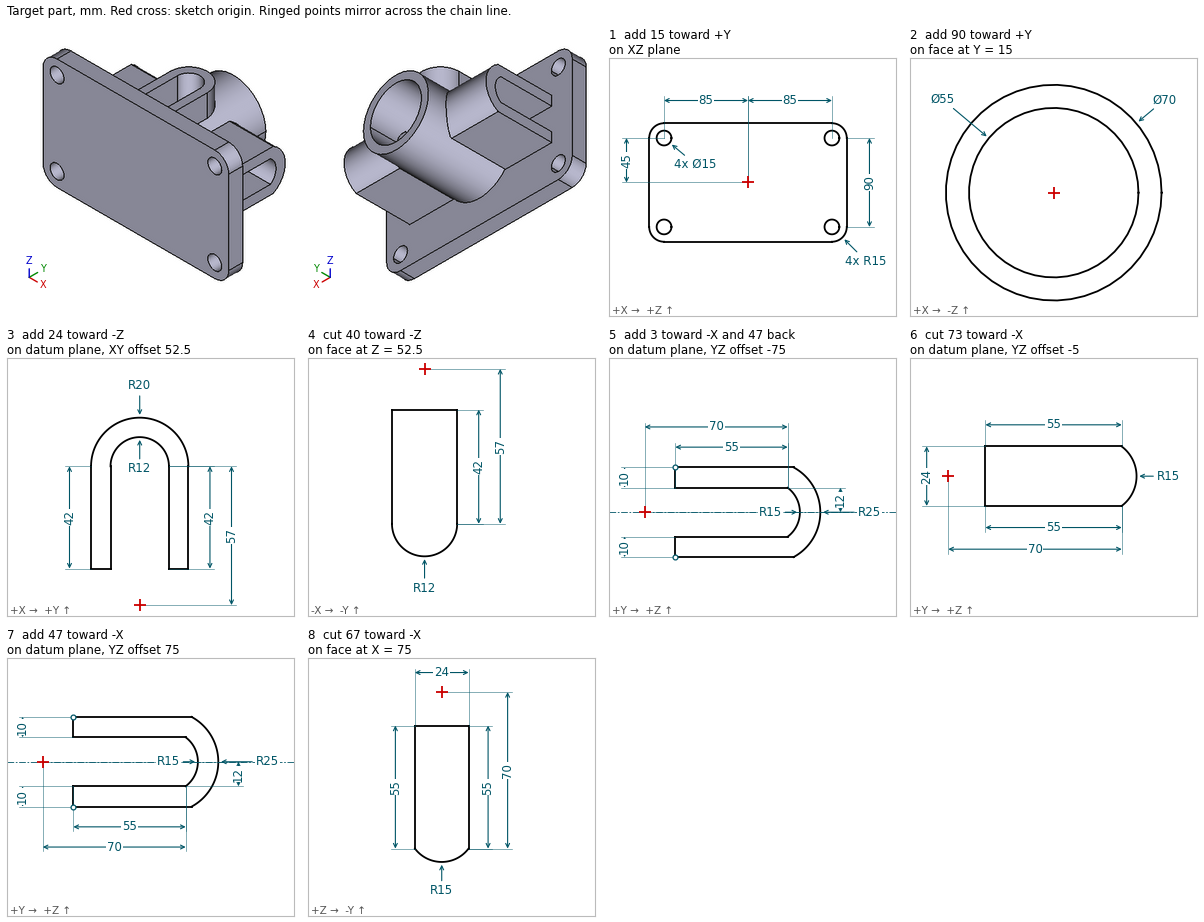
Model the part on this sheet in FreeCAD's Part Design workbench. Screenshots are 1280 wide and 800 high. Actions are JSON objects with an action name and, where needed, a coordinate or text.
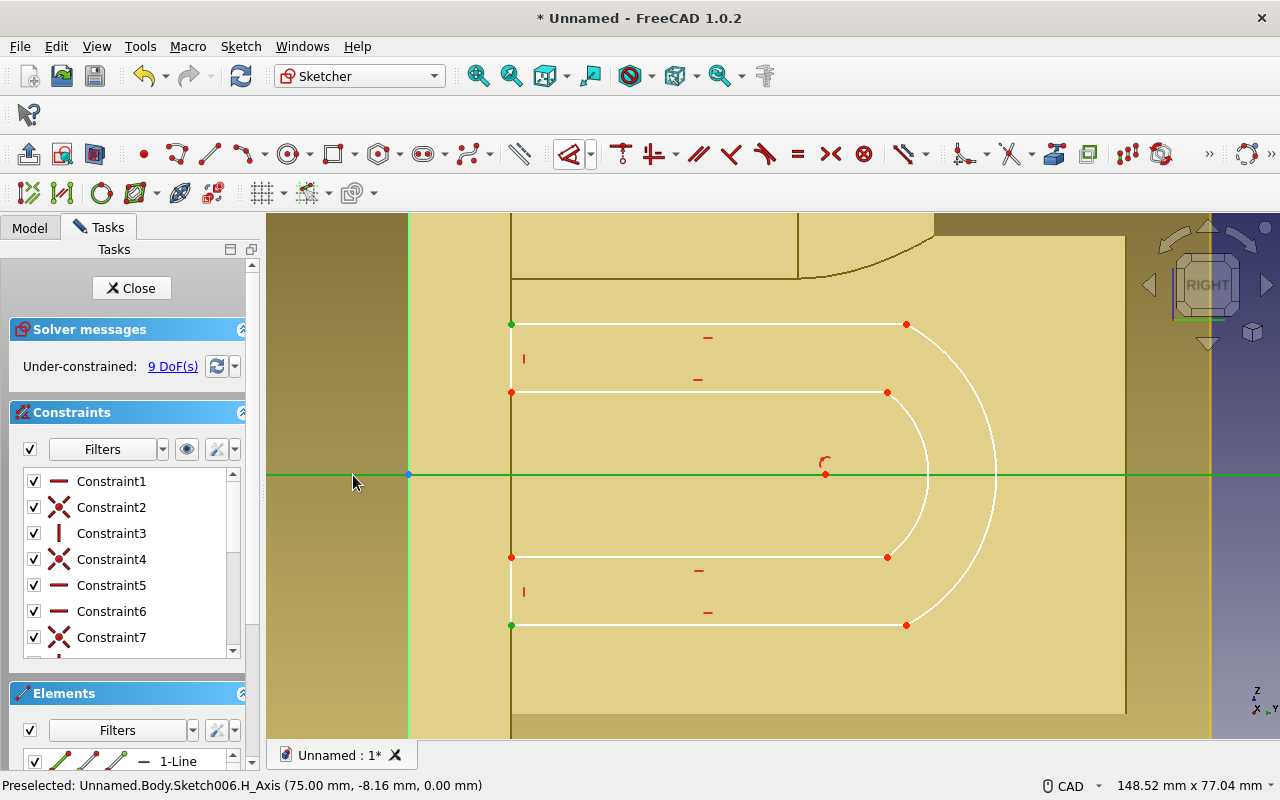
{"action": "key", "text": "s"}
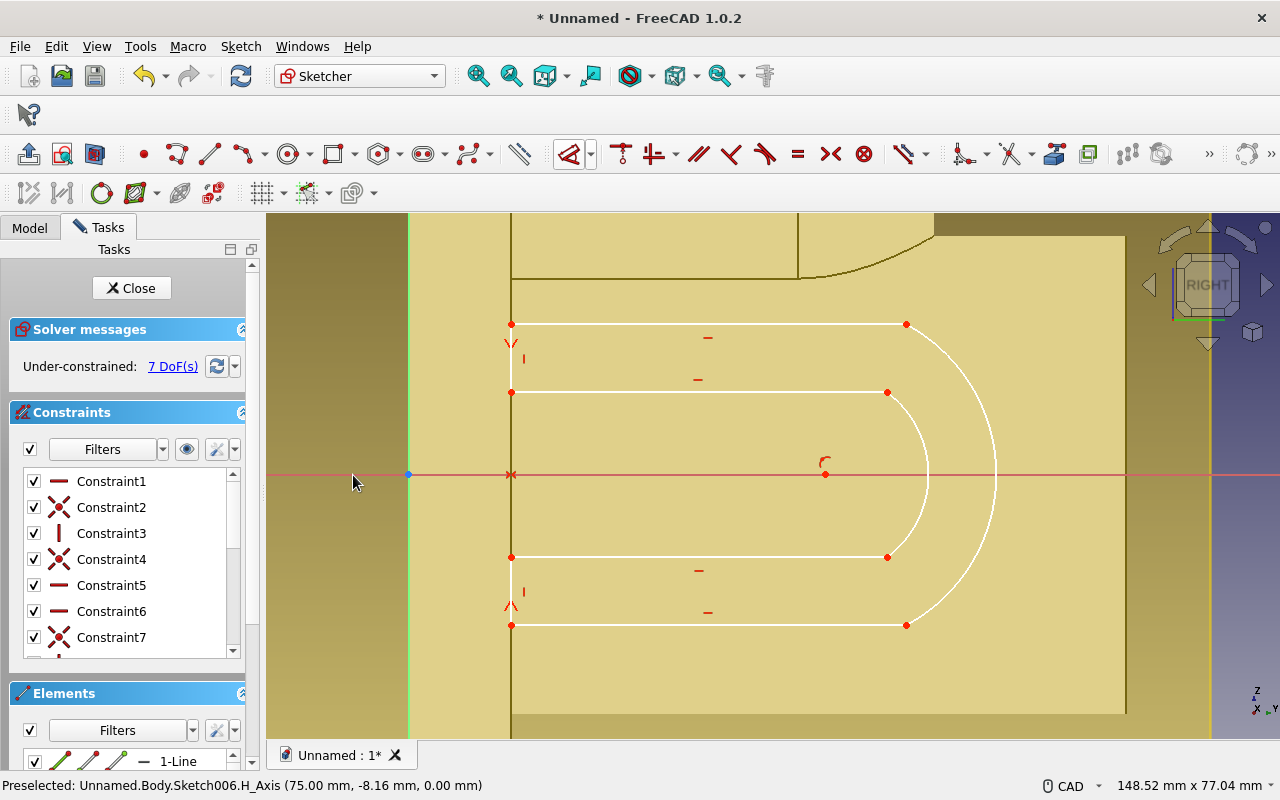
{"action": "left_click", "coordinate": [981, 546]}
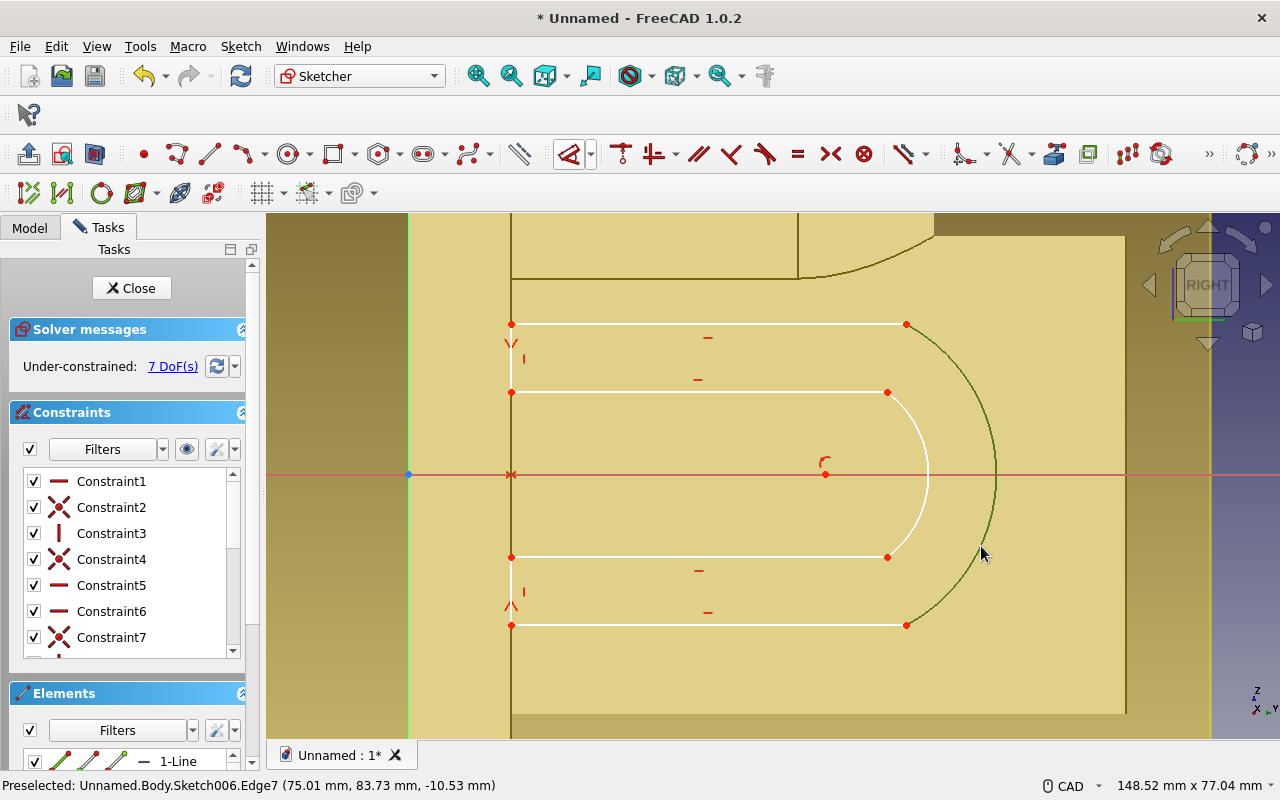
{"action": "left_click", "coordinate": [590, 154]}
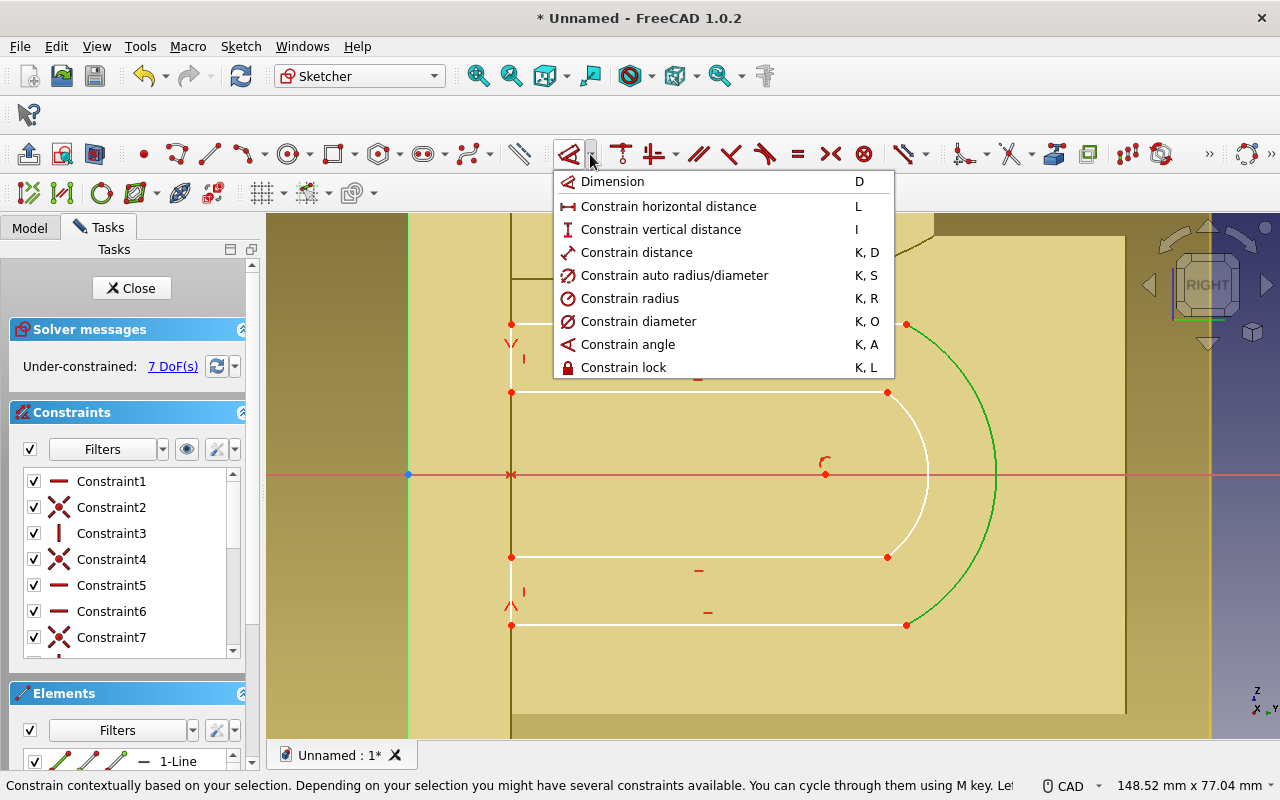
{"action": "left_click", "coordinate": [724, 298]}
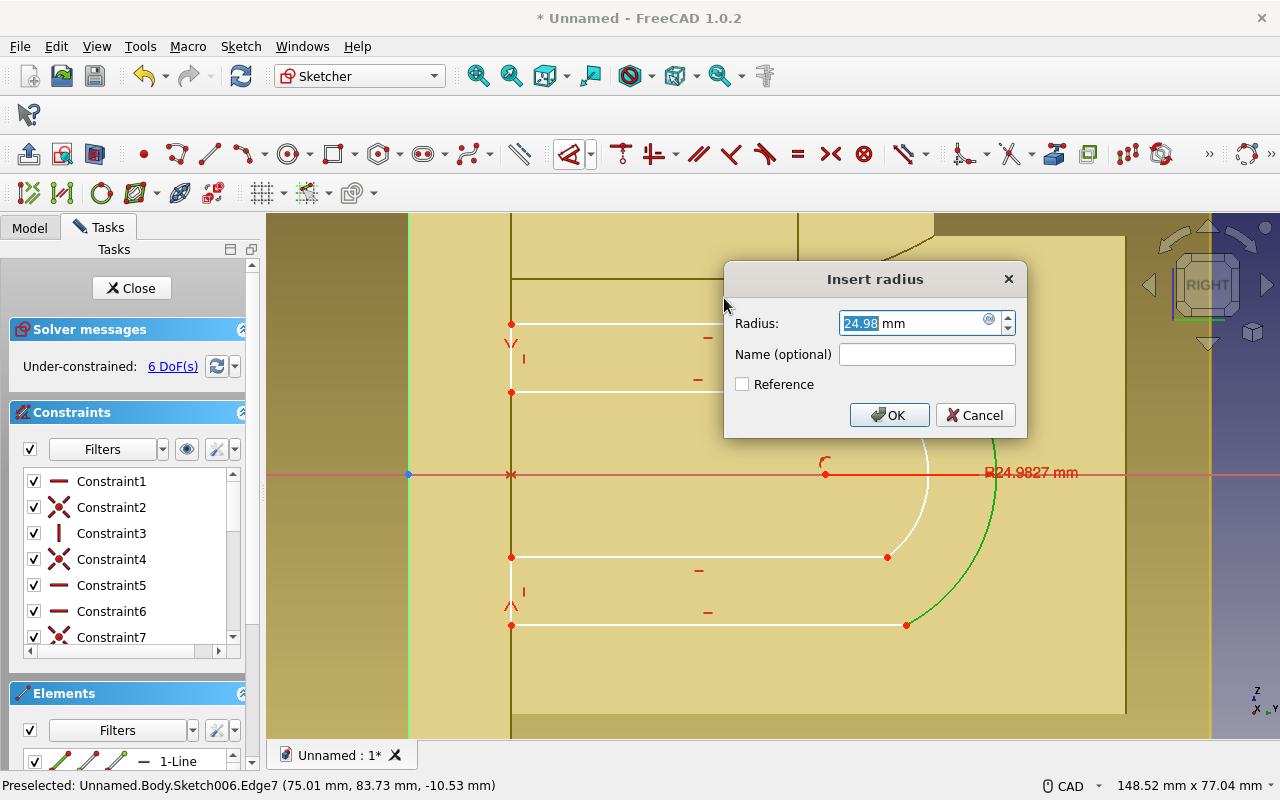
{"action": "type", "text": "25"}
{"action": "key", "text": "Return"}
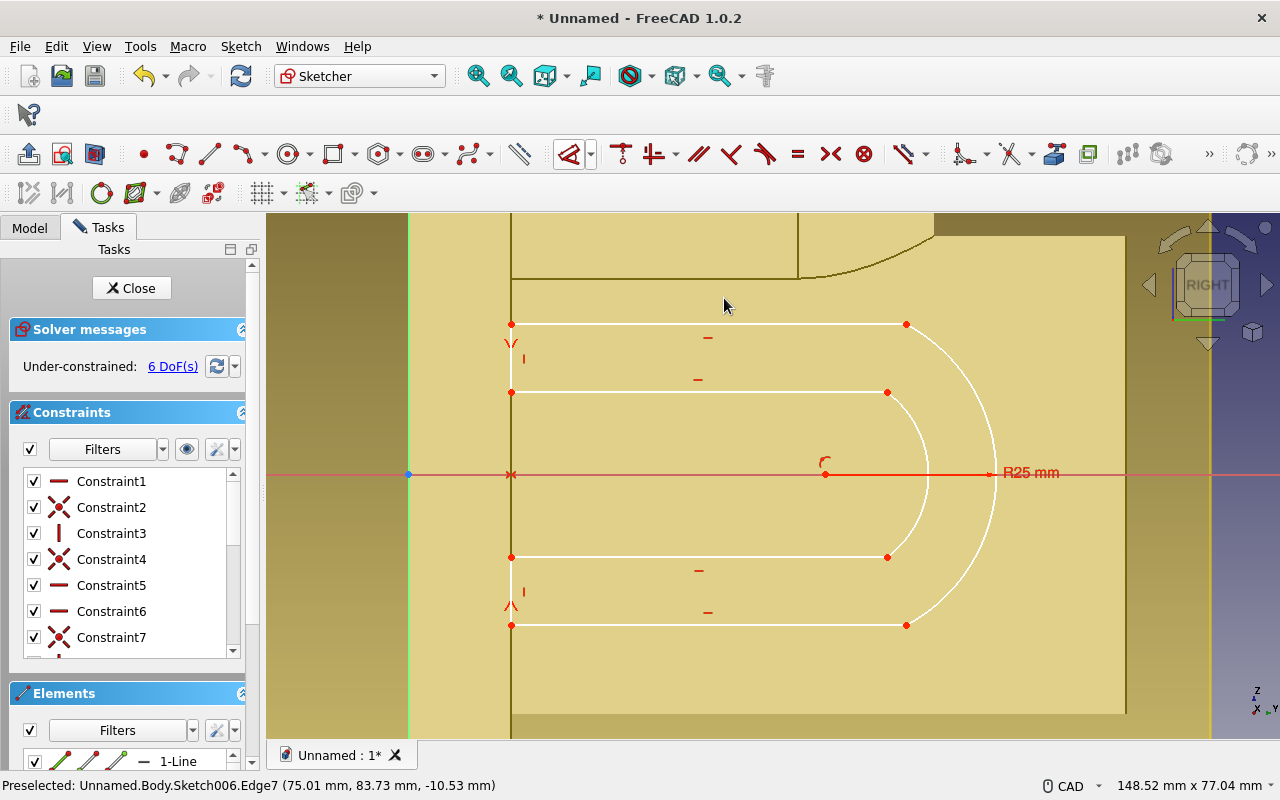
{"action": "left_click", "coordinate": [921, 512]}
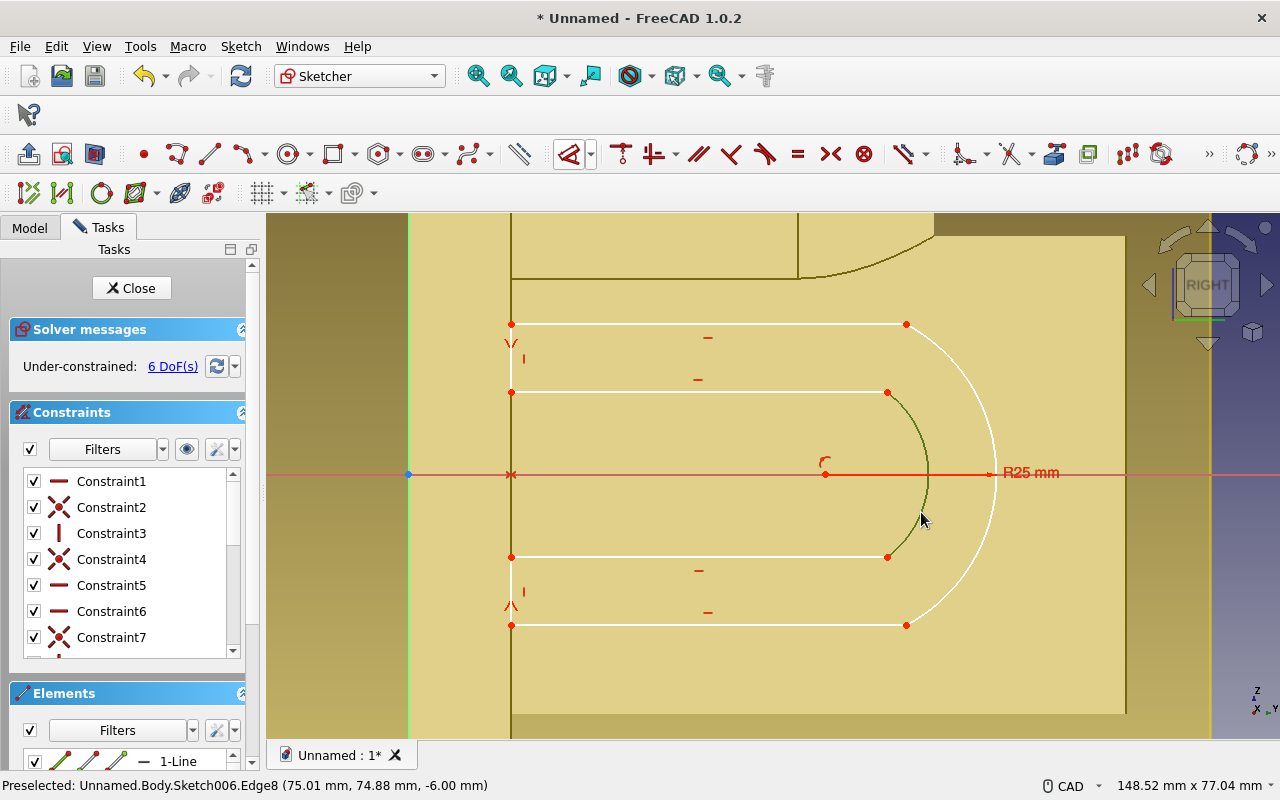
{"action": "key", "text": "k r"}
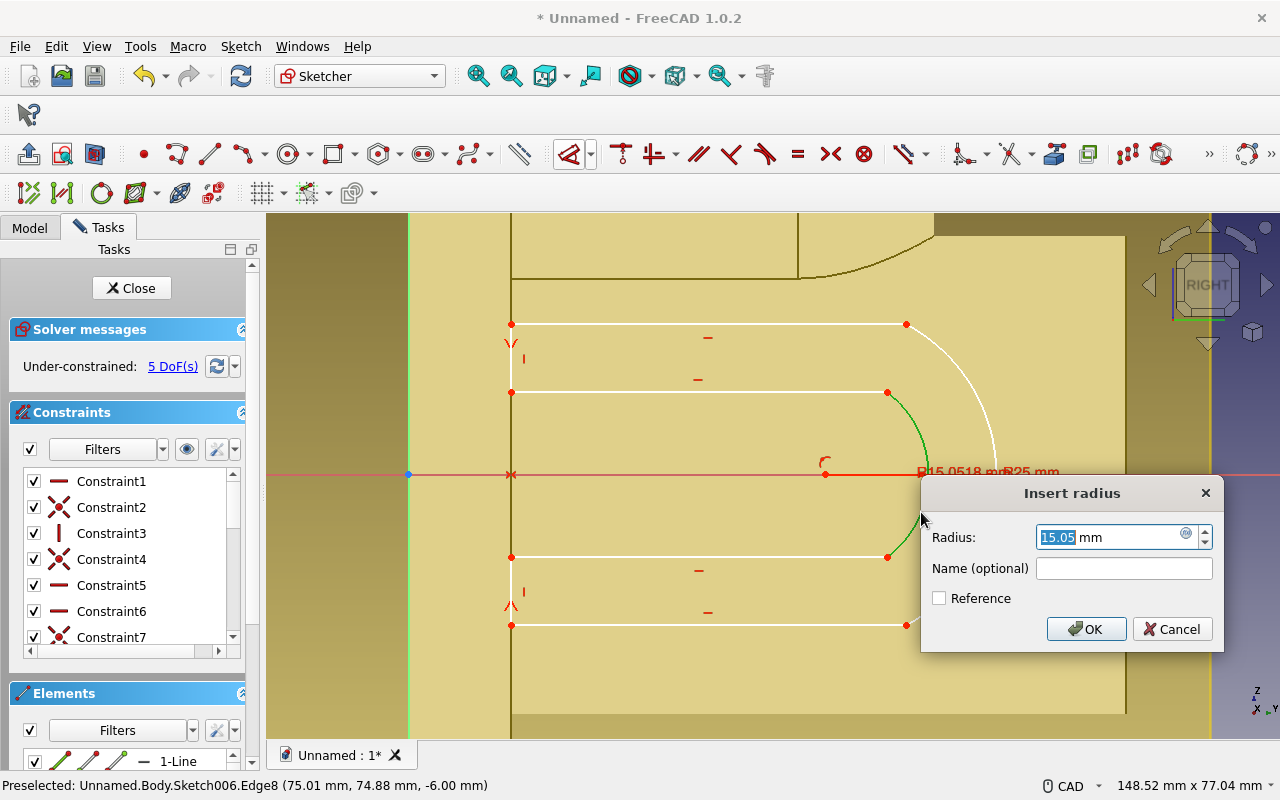
{"action": "type", "text": "15"}
{"action": "key", "text": "Return"}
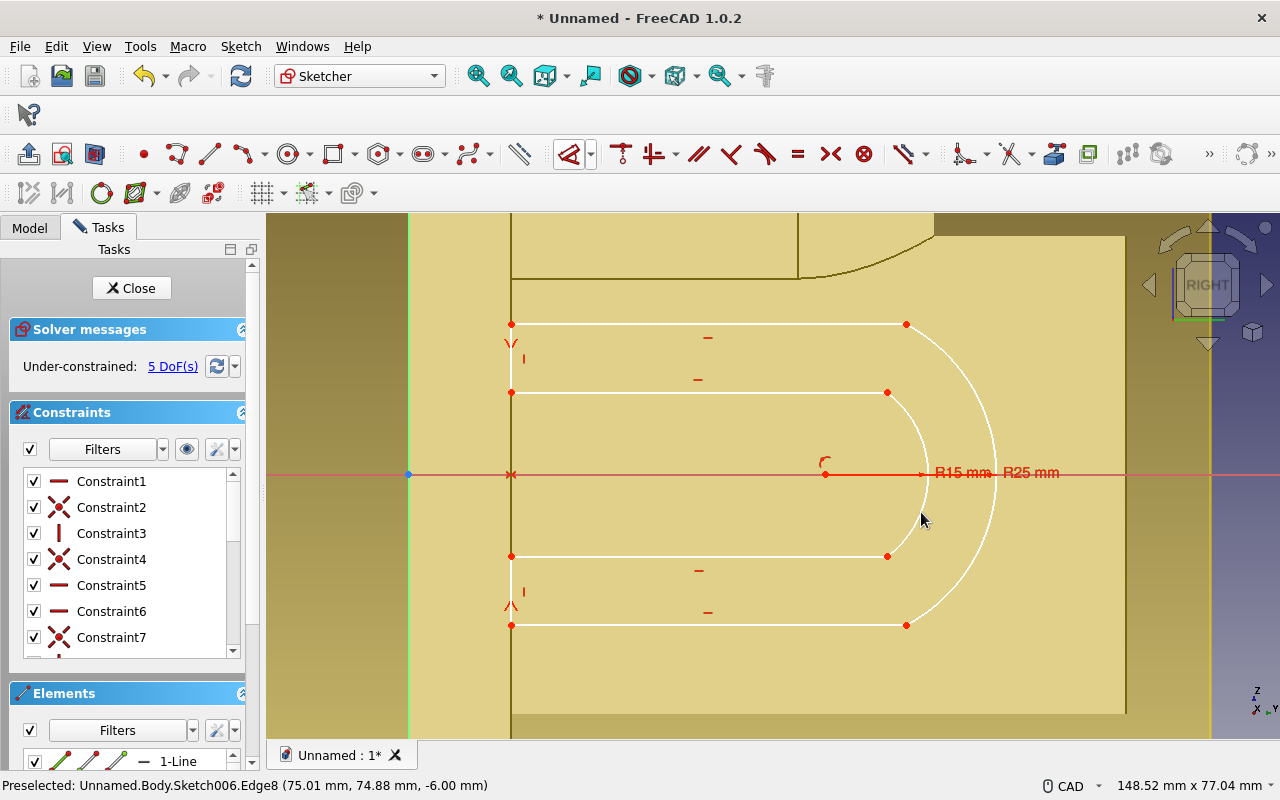
{"action": "left_click", "coordinate": [774, 557]}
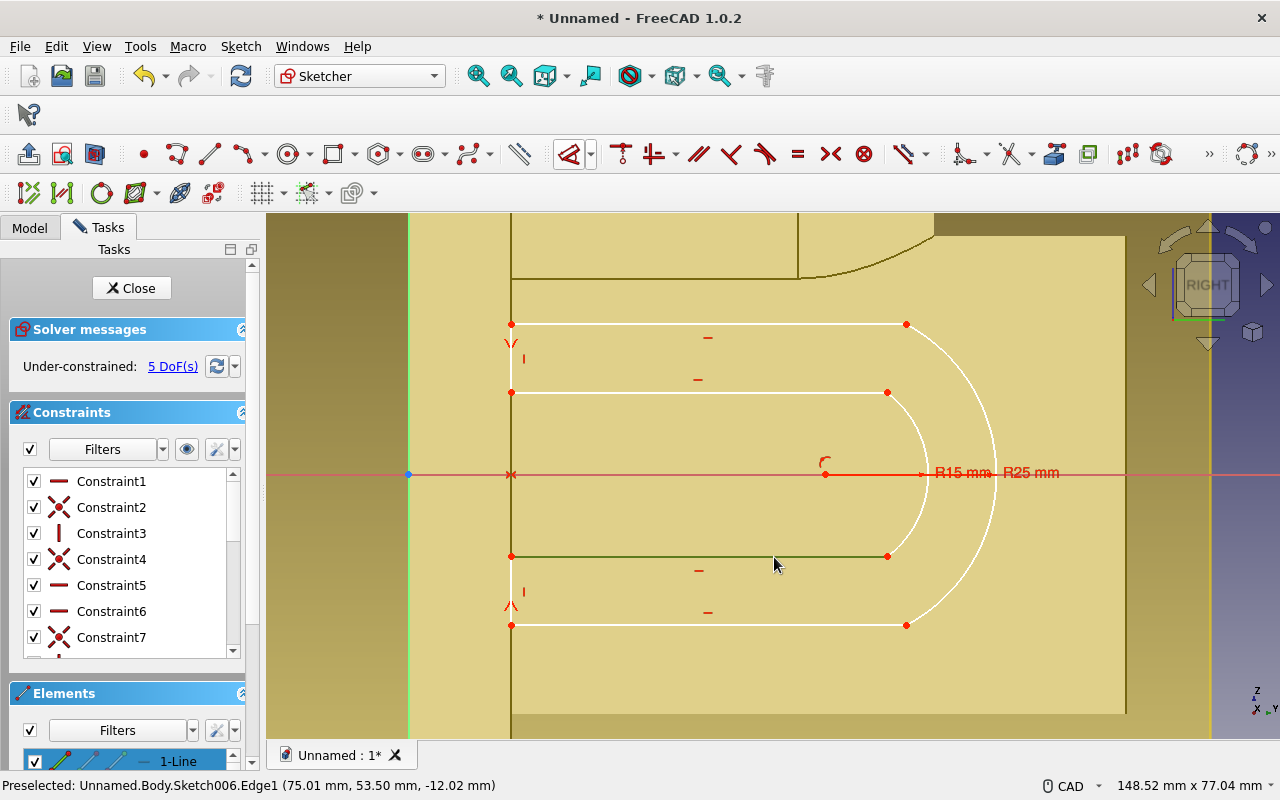
{"action": "key", "text": "l"}